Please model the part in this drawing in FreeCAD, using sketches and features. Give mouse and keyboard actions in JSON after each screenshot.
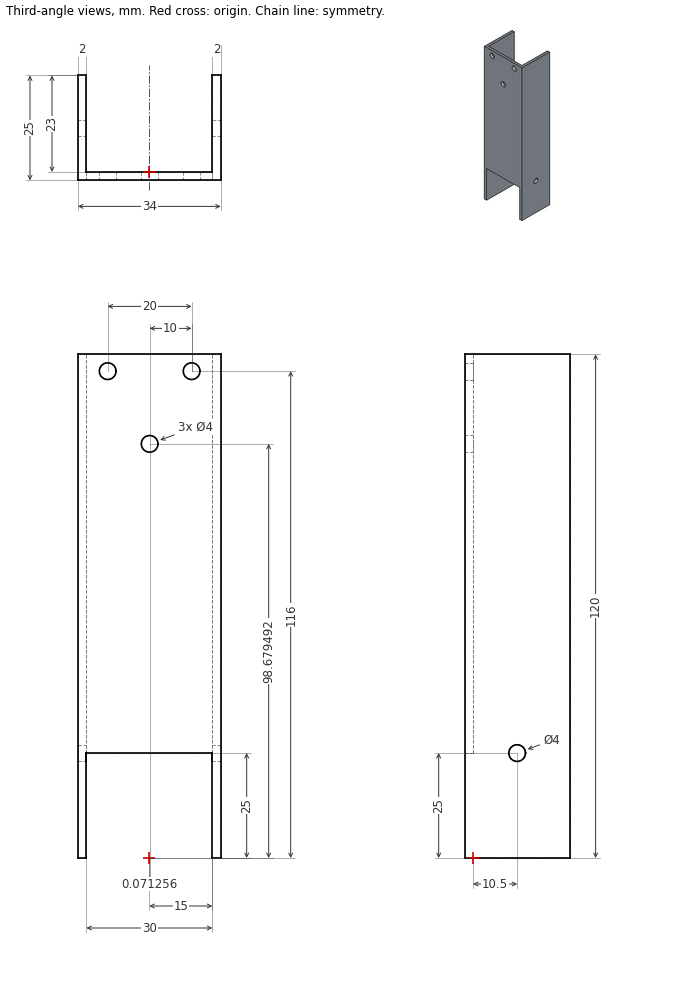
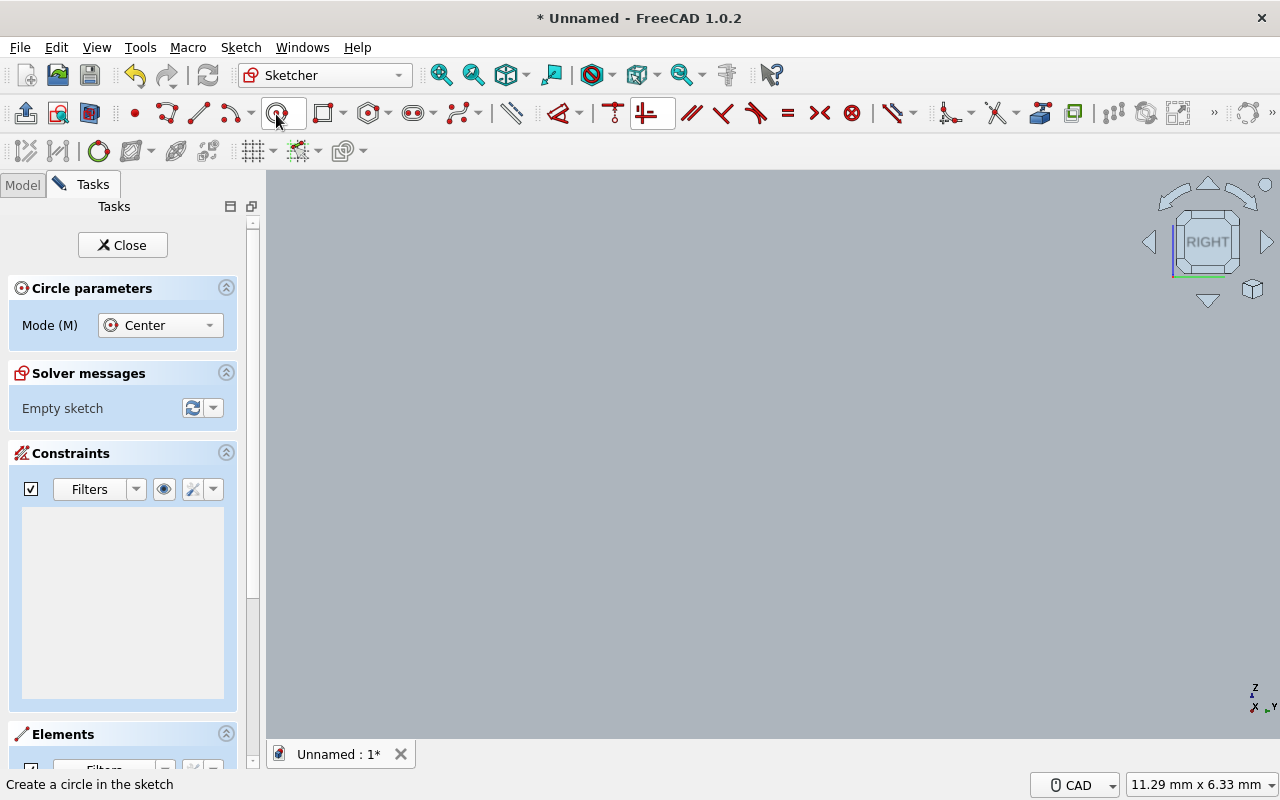
{"action": "left_click", "coordinate": [687, 444]}
{"action": "left_click", "coordinate": [814, 317]}
{"action": "key", "text": "Escape"}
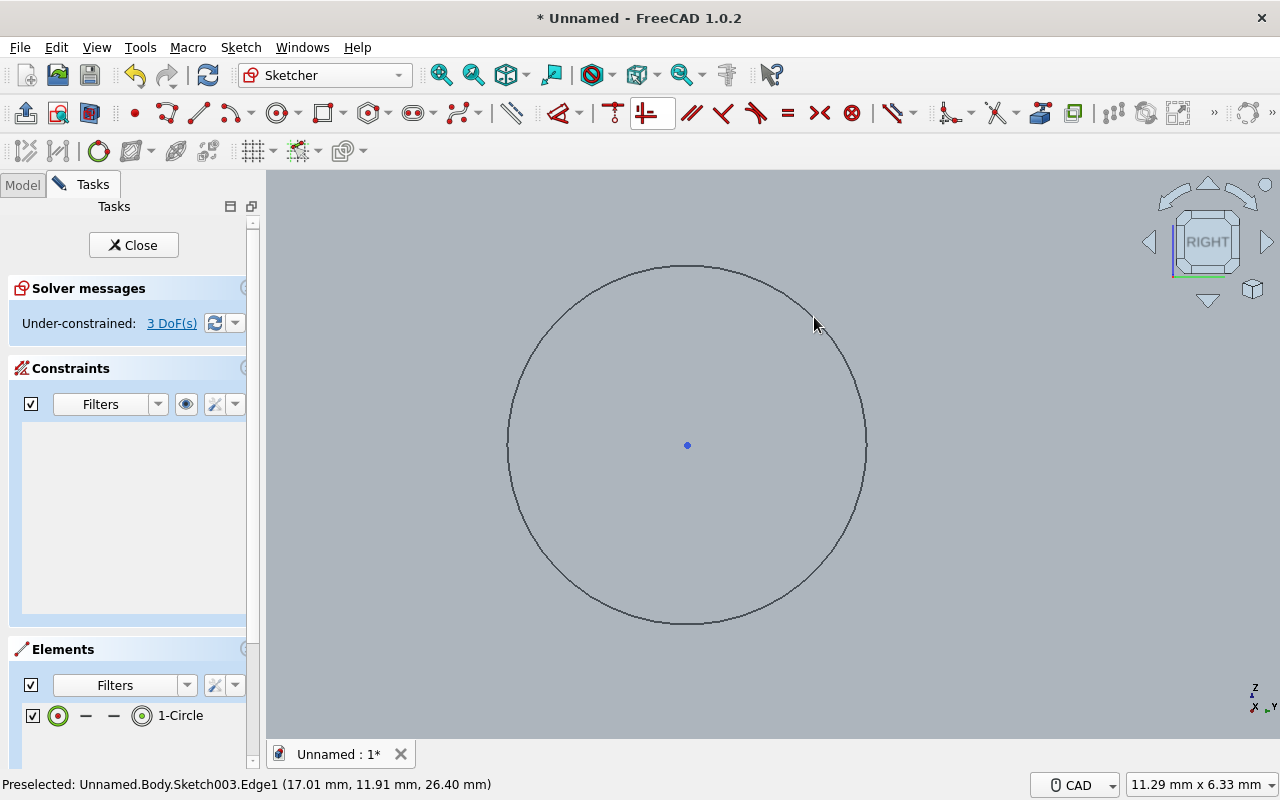
{"action": "left_click", "coordinate": [558, 114]}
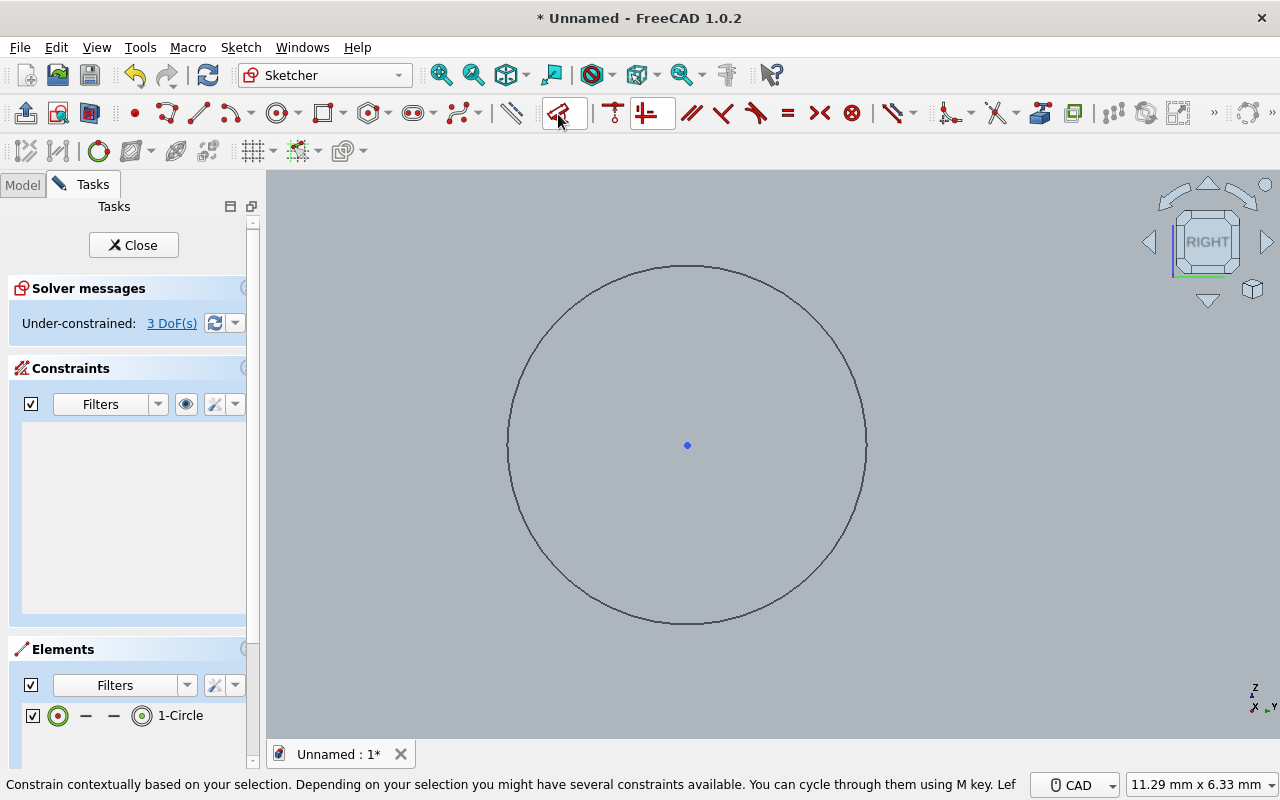
{"action": "left_click", "coordinate": [814, 318]}
{"action": "left_click", "coordinate": [837, 295]}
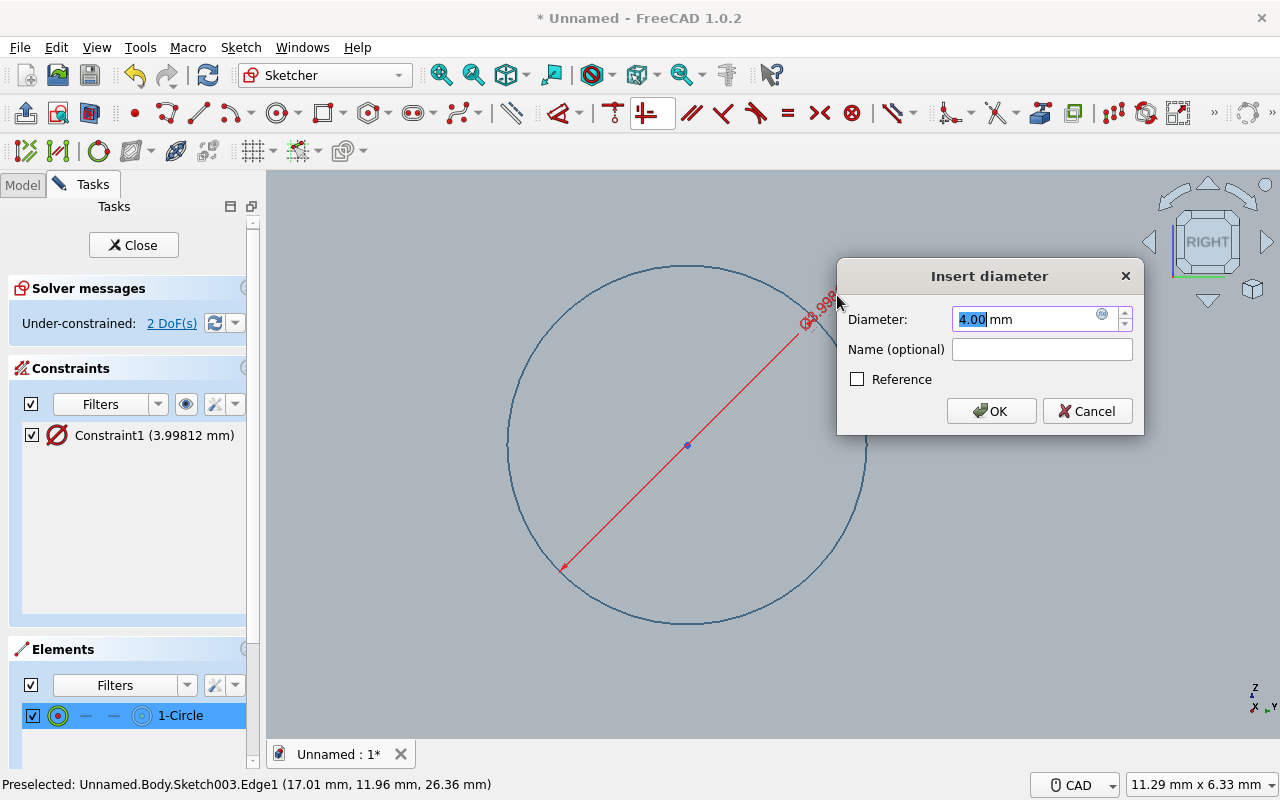
{"action": "type", "text": "4"}
{"action": "key", "text": "Return"}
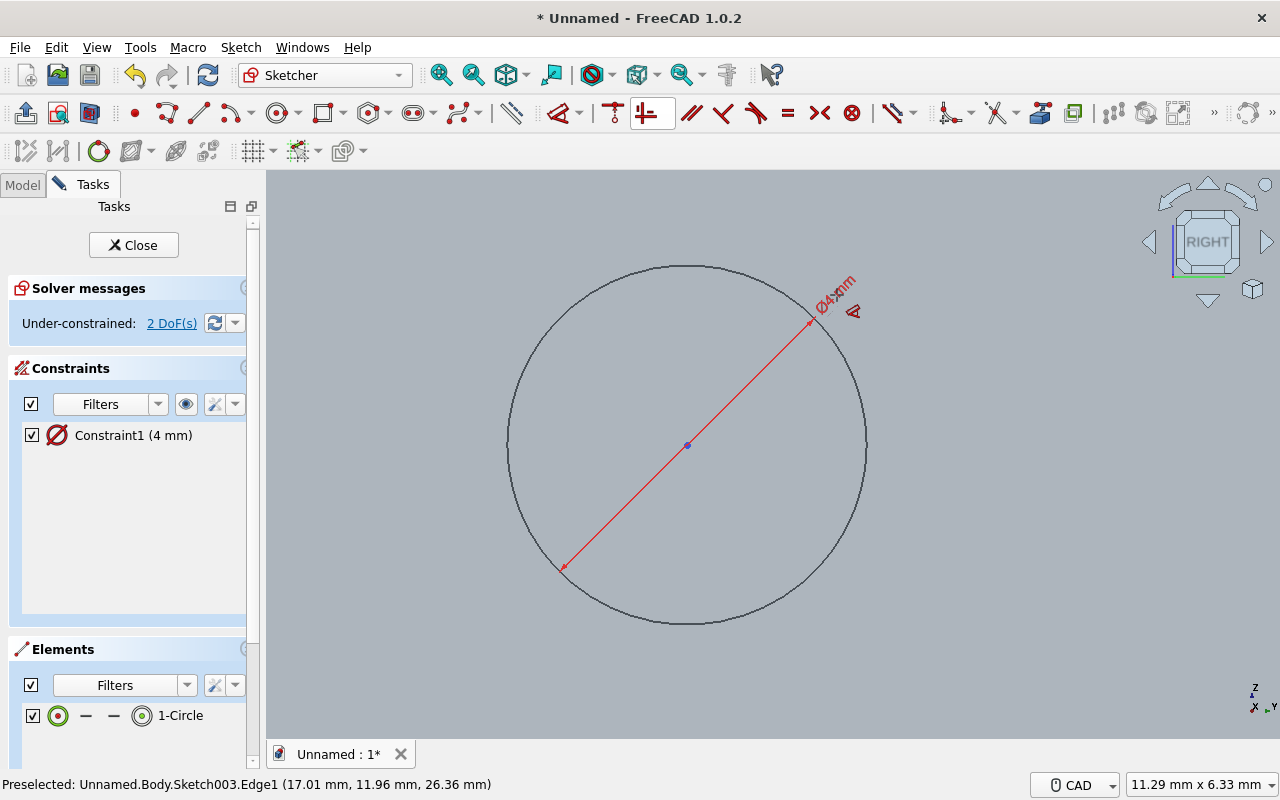
{"action": "left_click", "coordinate": [687, 445]}
{"action": "left_click", "coordinate": [721, 578]}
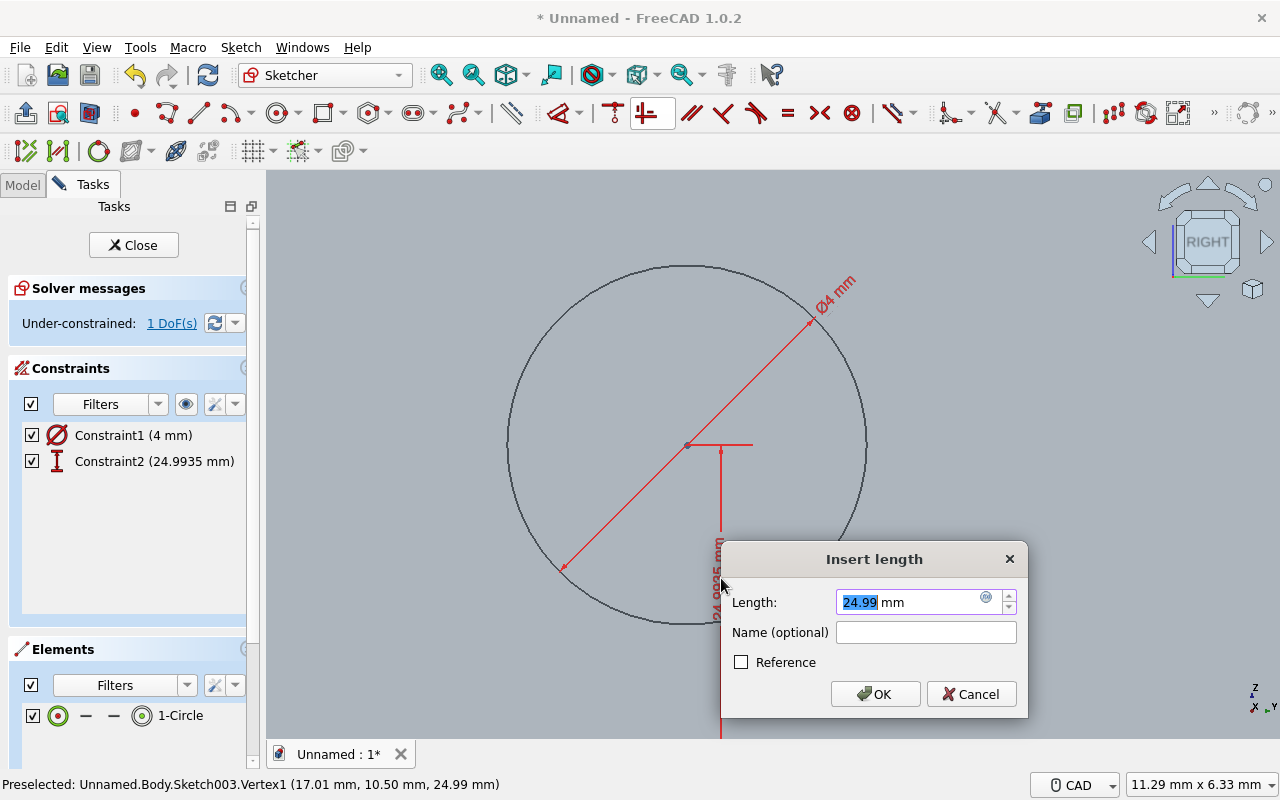
{"action": "type", "text": "25"}
{"action": "key", "text": "Return"}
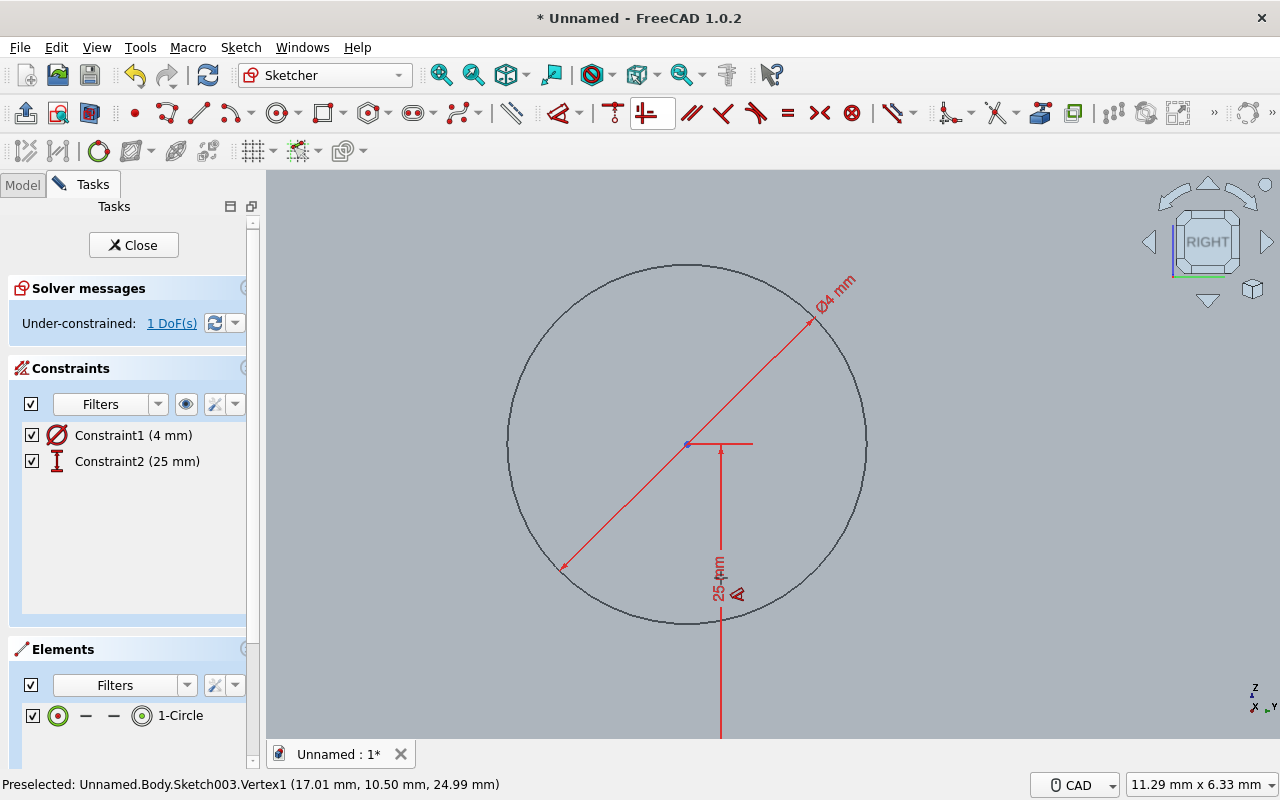
{"action": "left_click", "coordinate": [687, 444]}
{"action": "left_click", "coordinate": [491, 410]}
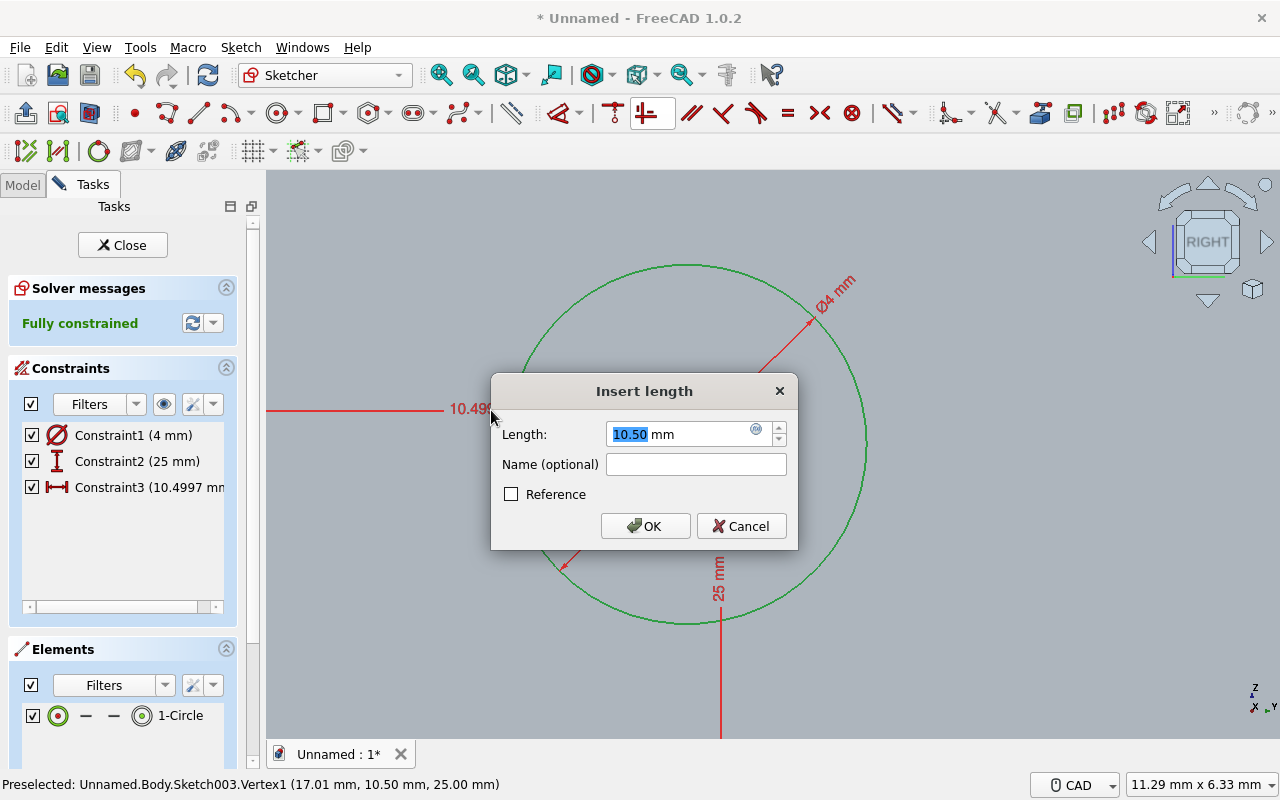
{"action": "type", "text": "10.5"}
{"action": "key", "text": "Return"}
{"action": "key", "text": "Escape"}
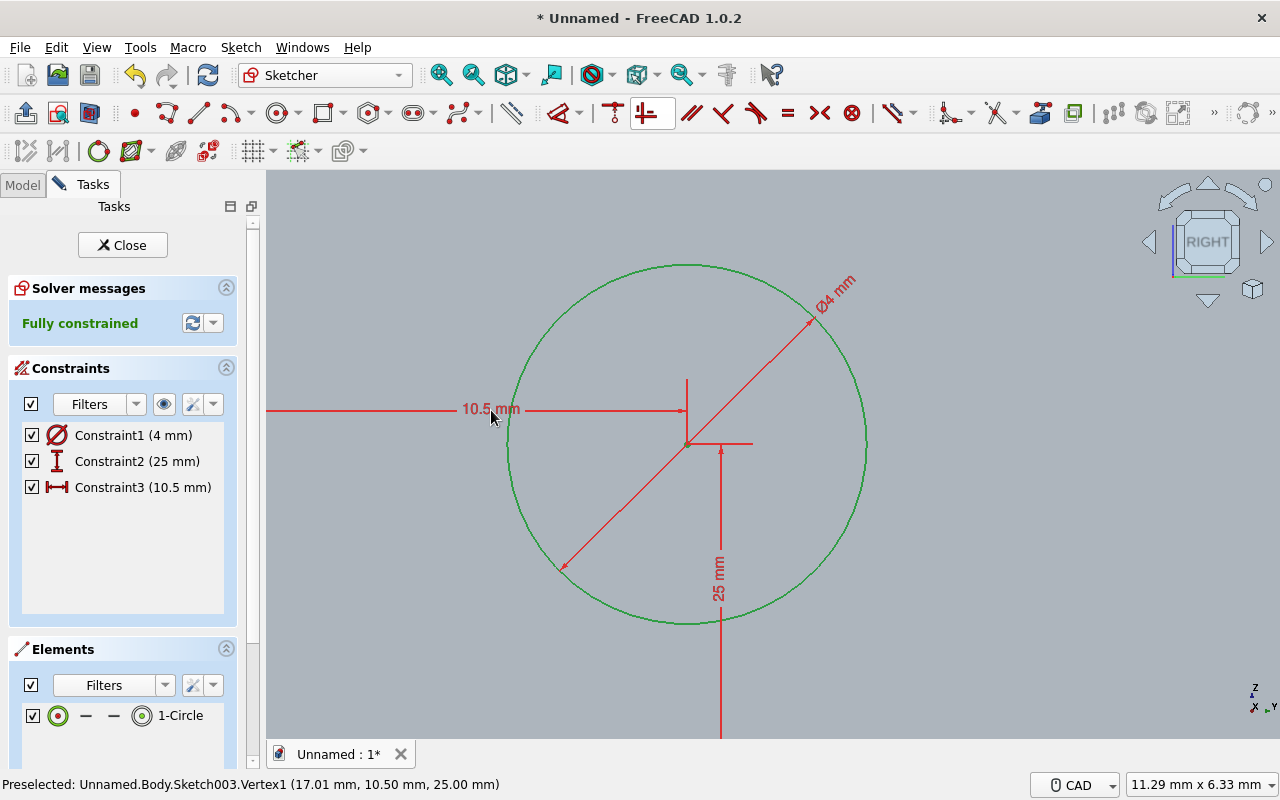
{"action": "left_click", "coordinate": [123, 245]}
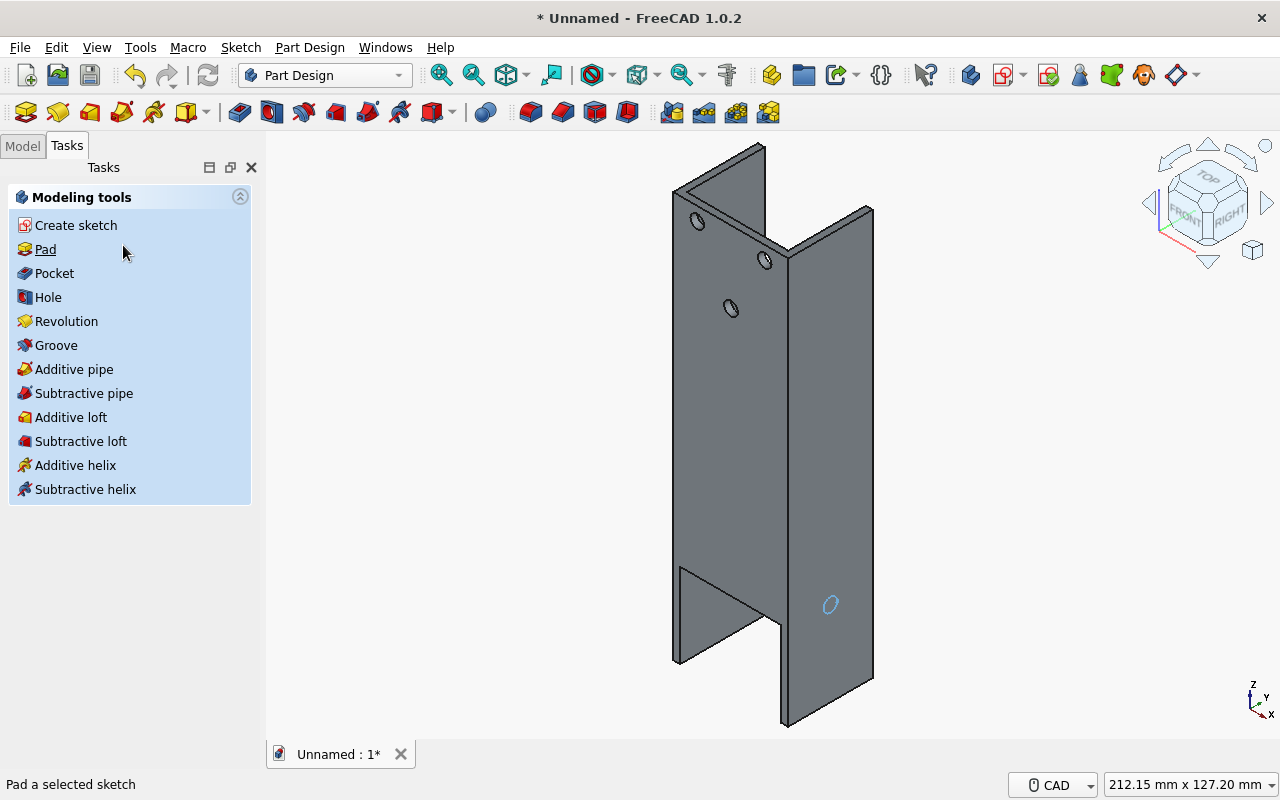
{"action": "left_click", "coordinate": [240, 112]}